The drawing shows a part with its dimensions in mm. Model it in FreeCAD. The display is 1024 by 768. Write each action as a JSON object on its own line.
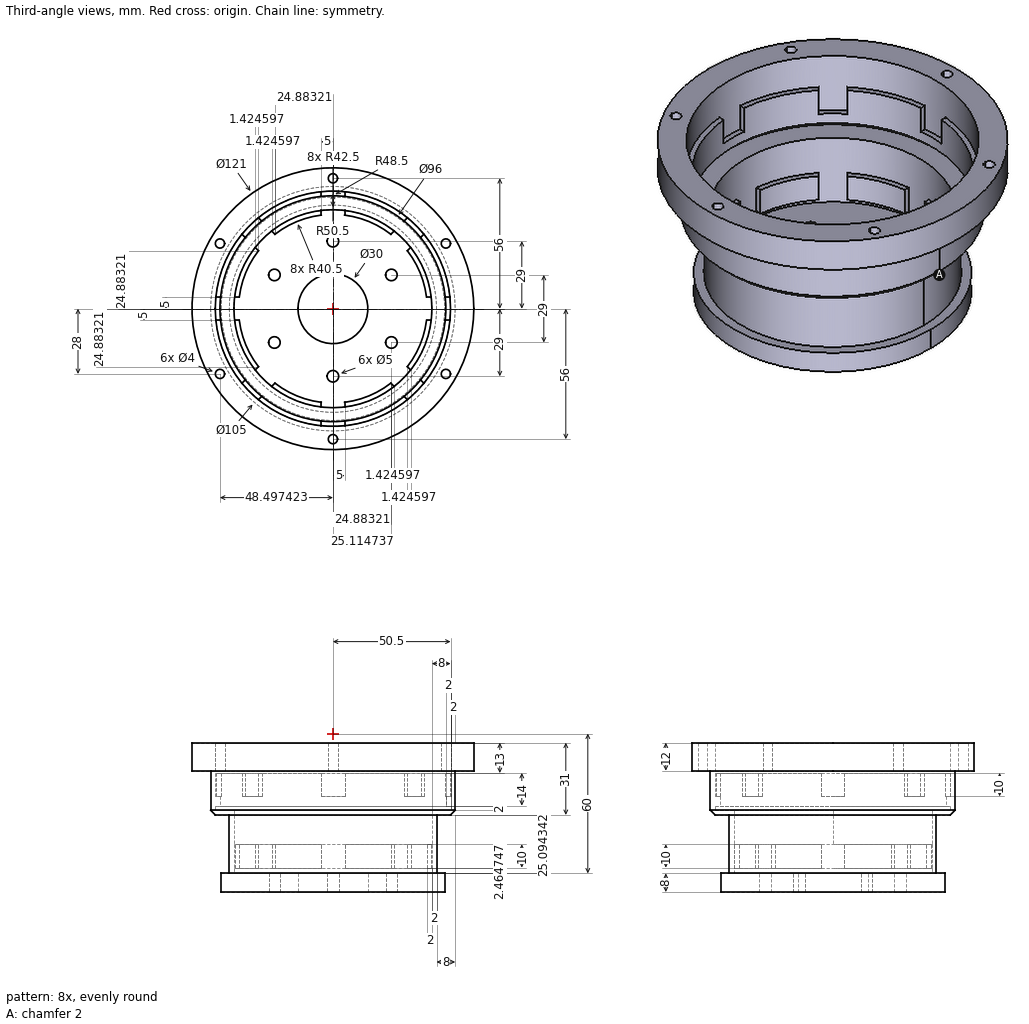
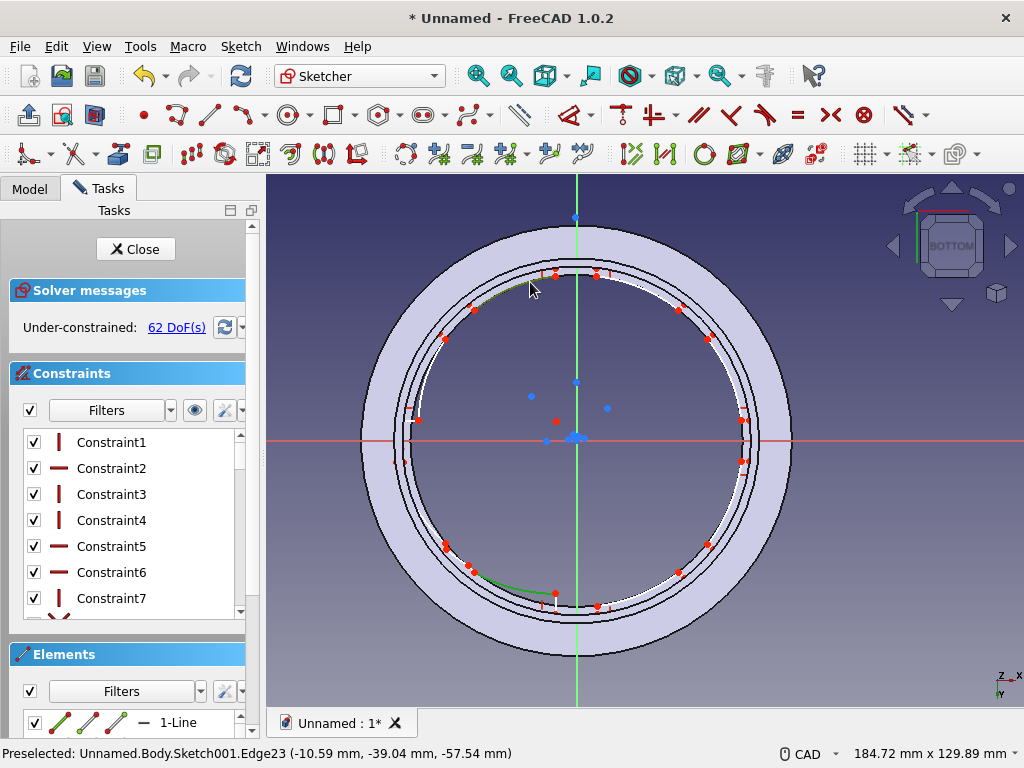
{"action": "left_click", "coordinate": [621, 116]}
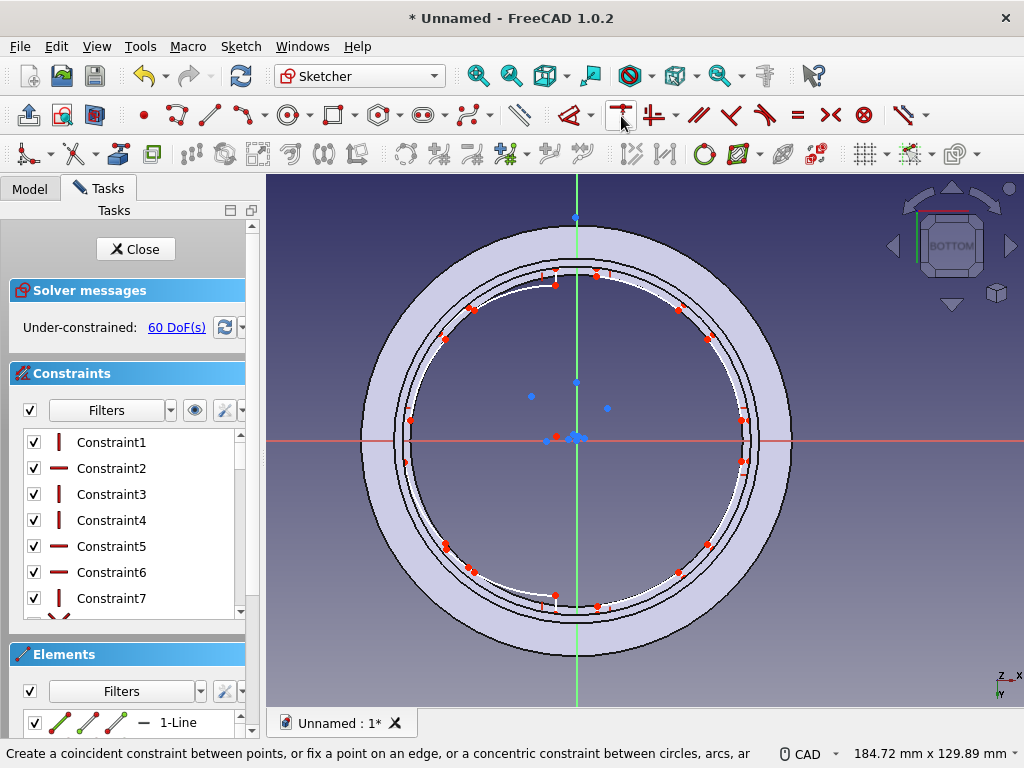
{"action": "left_click", "coordinate": [497, 584]}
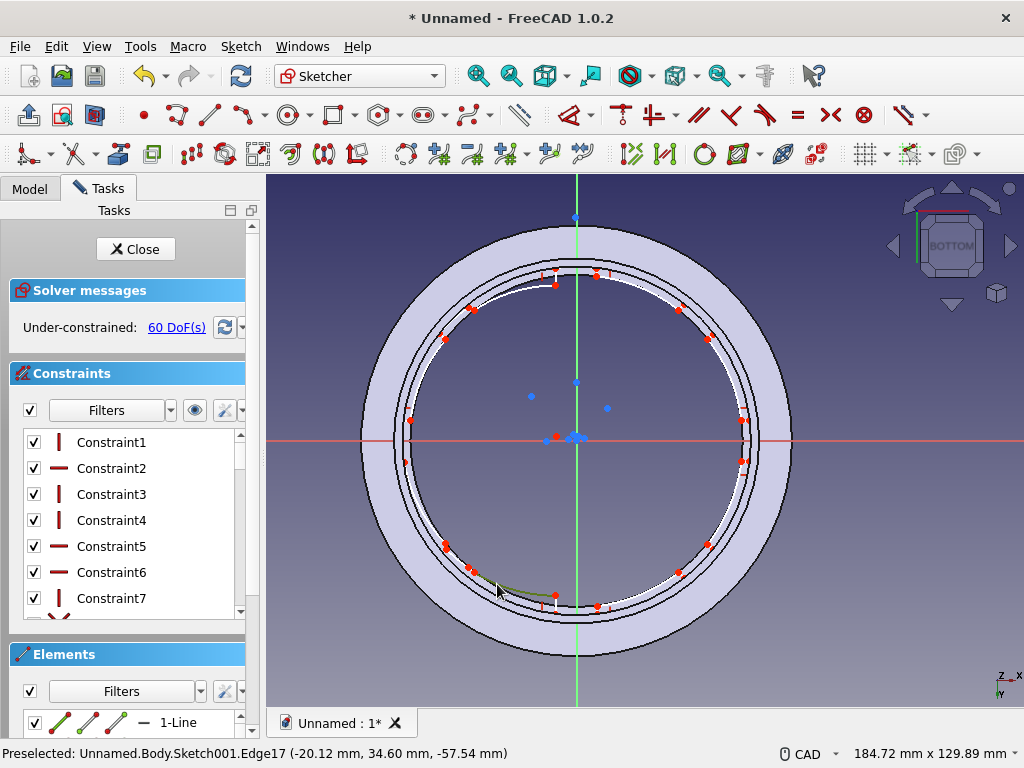
{"action": "left_click", "coordinate": [576, 267]}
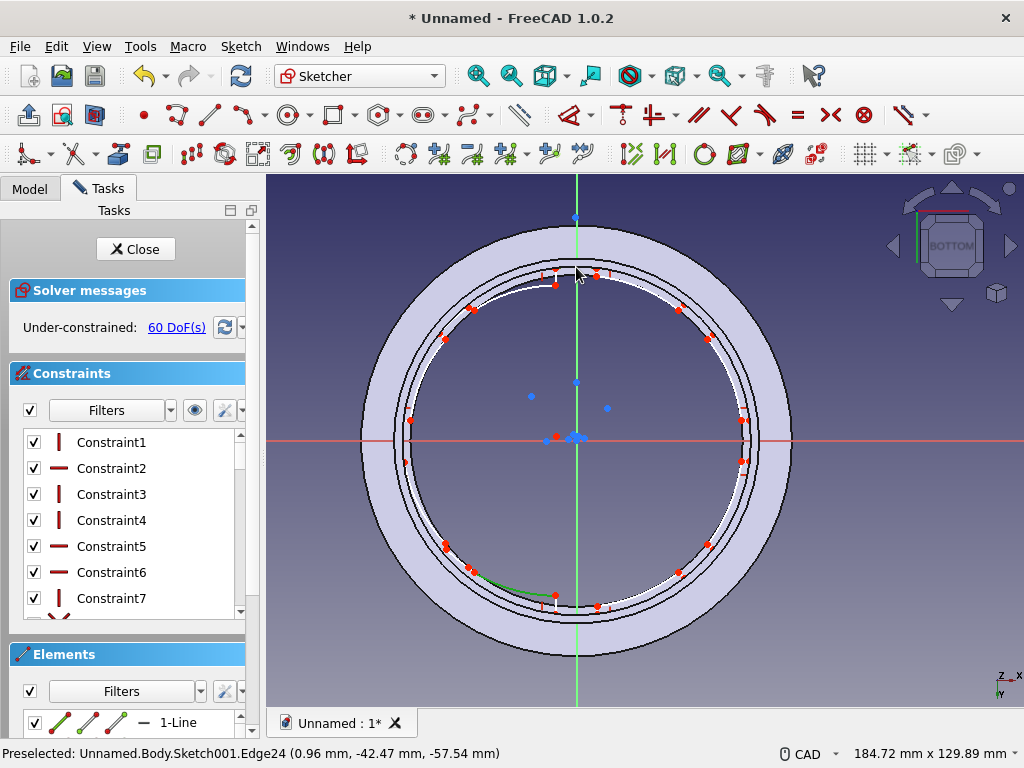
{"action": "left_click", "coordinate": [621, 116]}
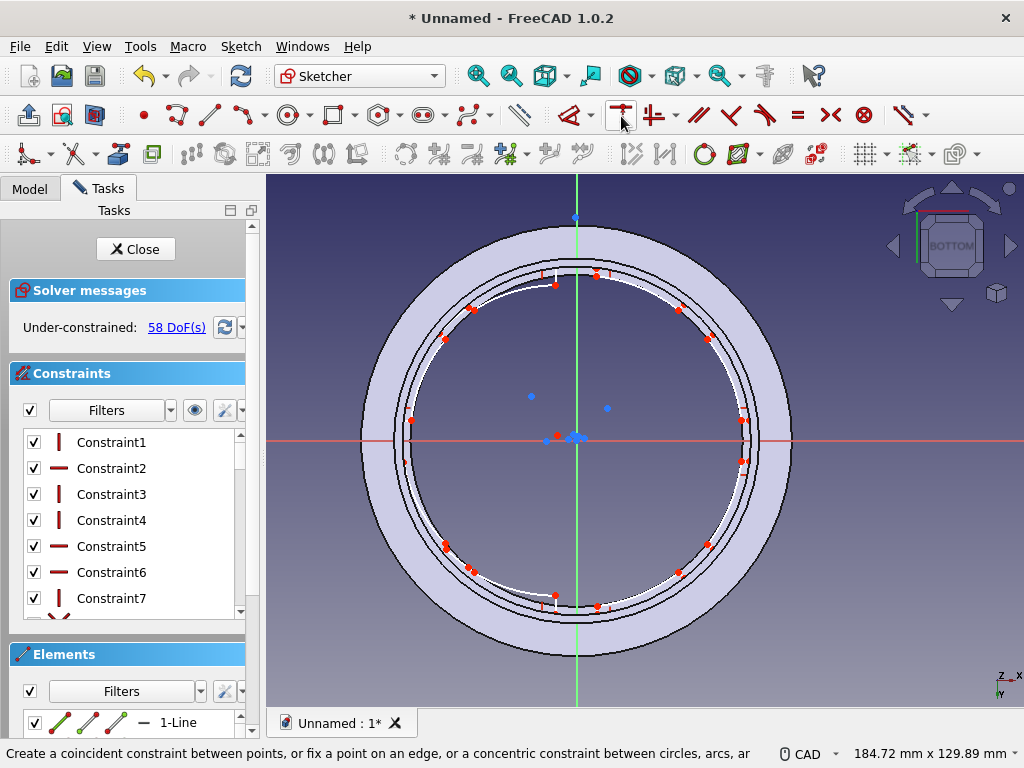
{"action": "left_click", "coordinate": [497, 584]}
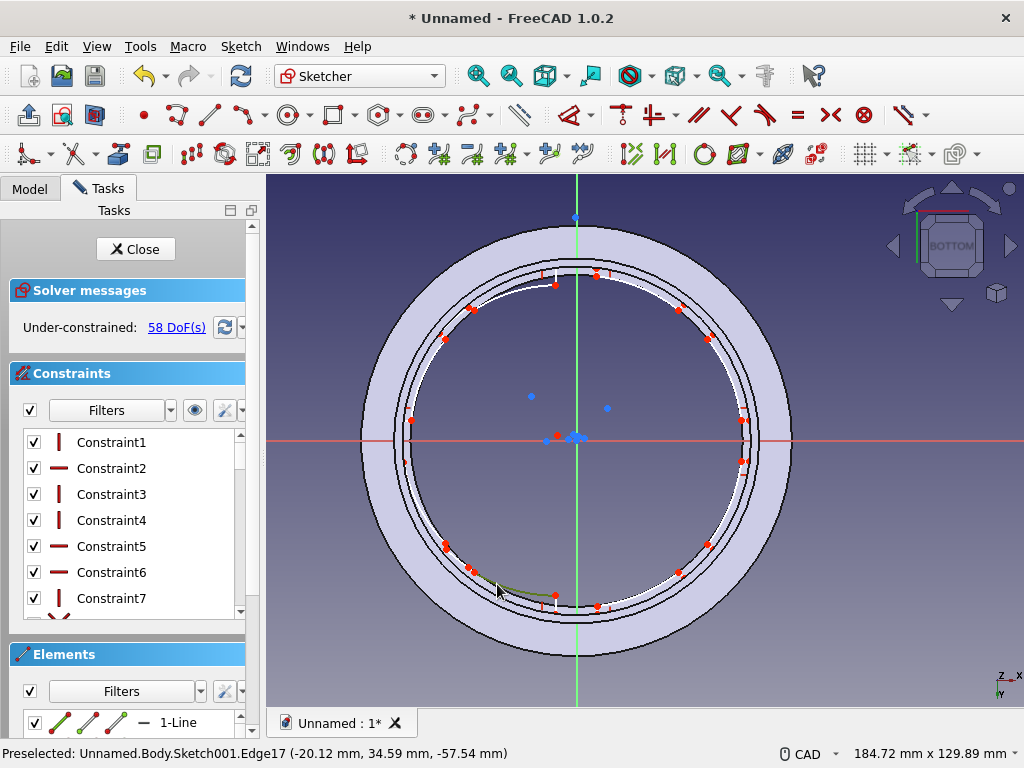
{"action": "left_click", "coordinate": [656, 295]}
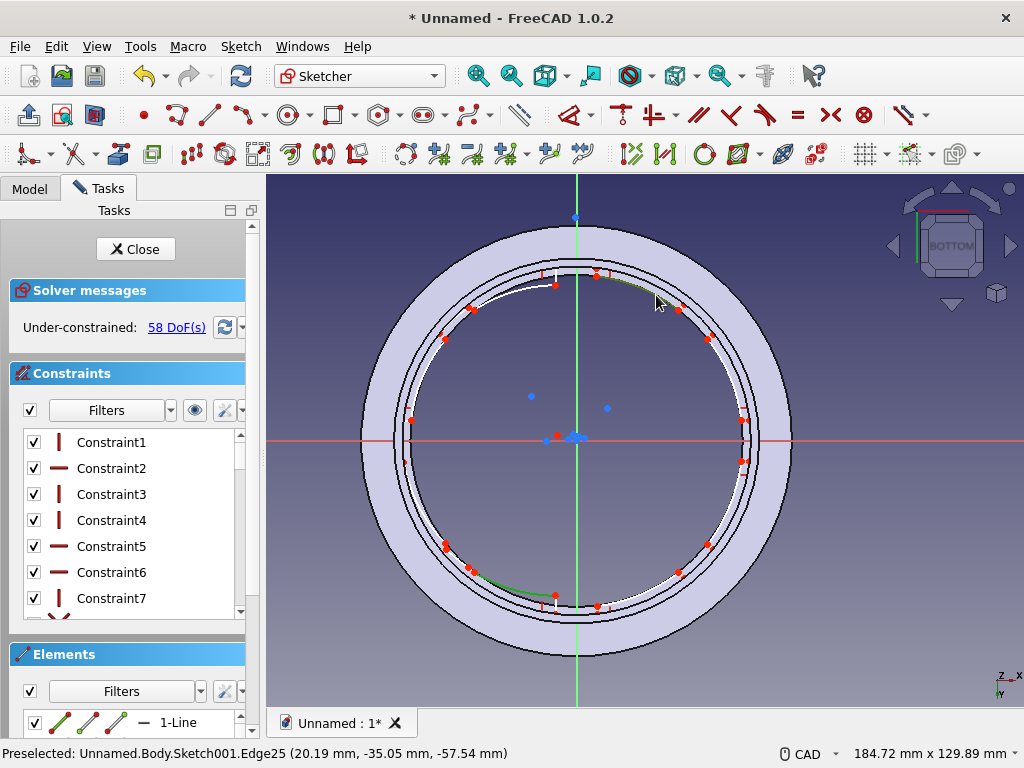
{"action": "key", "text": "c"}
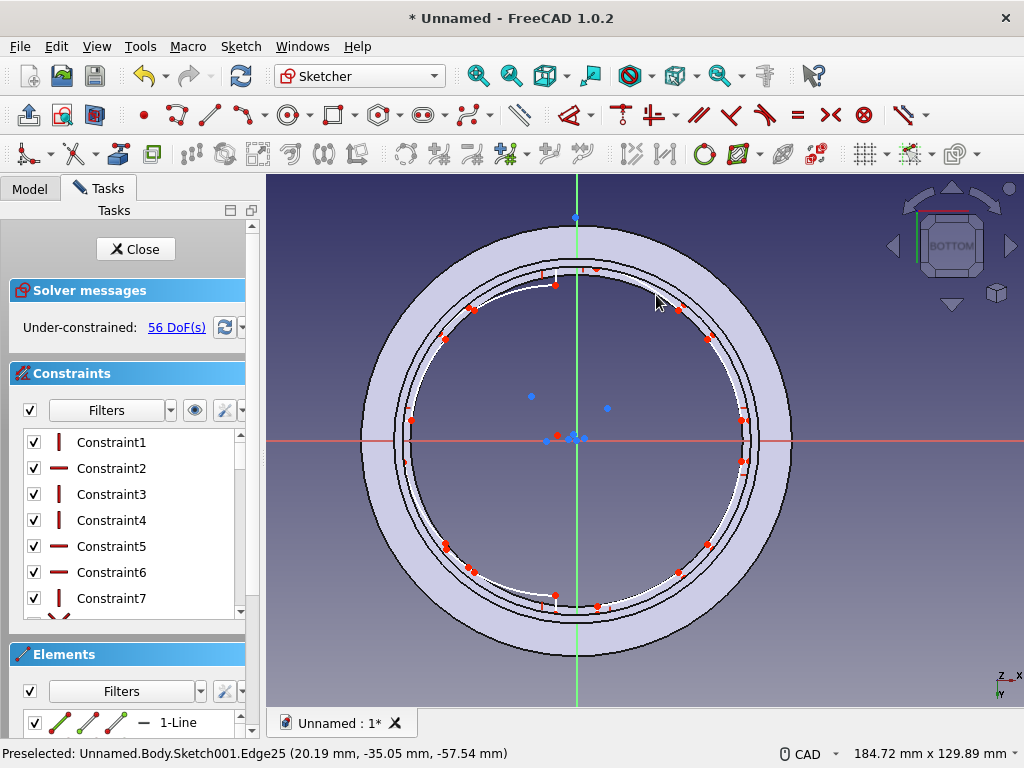
{"action": "left_click", "coordinate": [497, 584]}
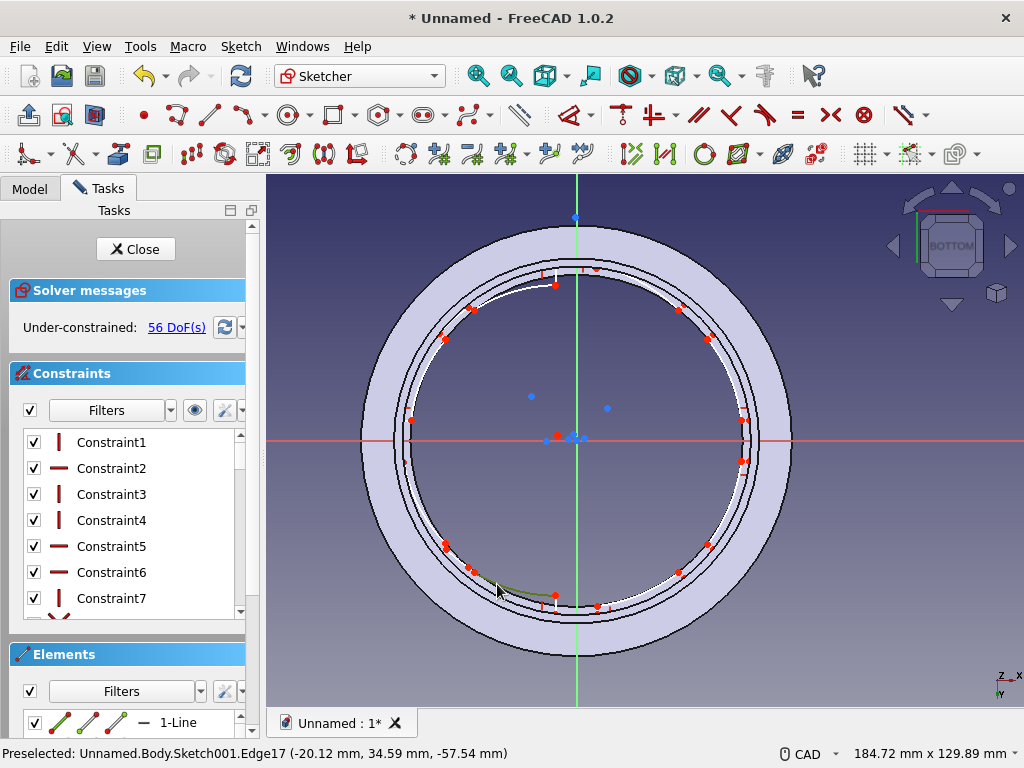
{"action": "left_click", "coordinate": [706, 324]}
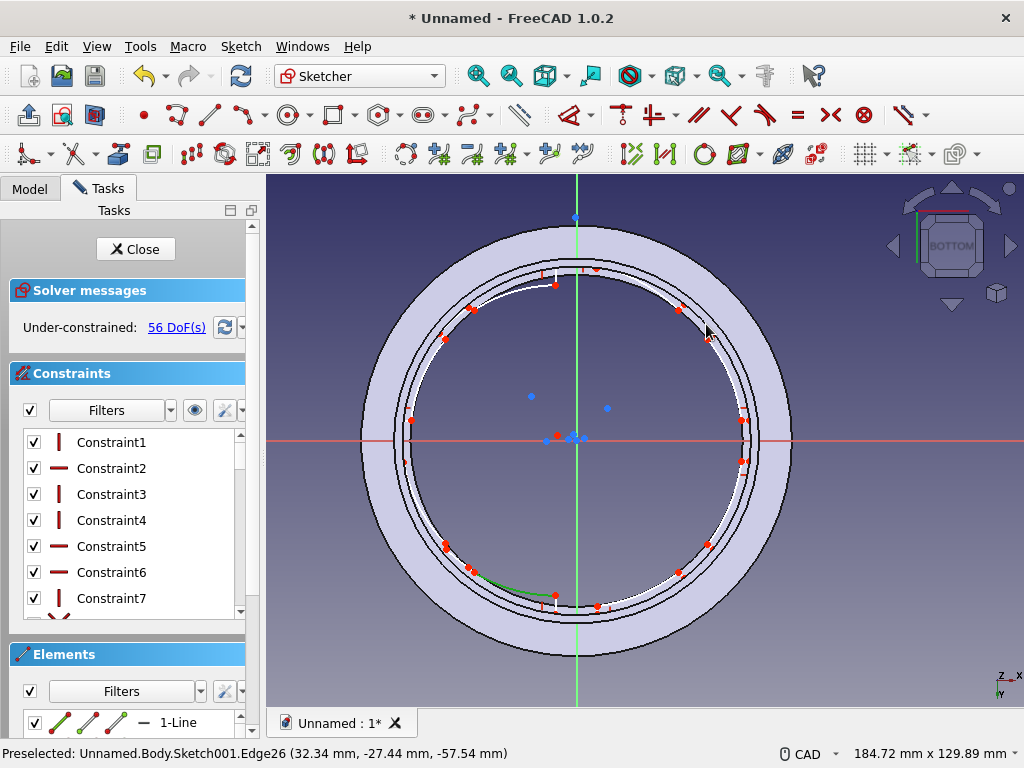
{"action": "key", "text": "c"}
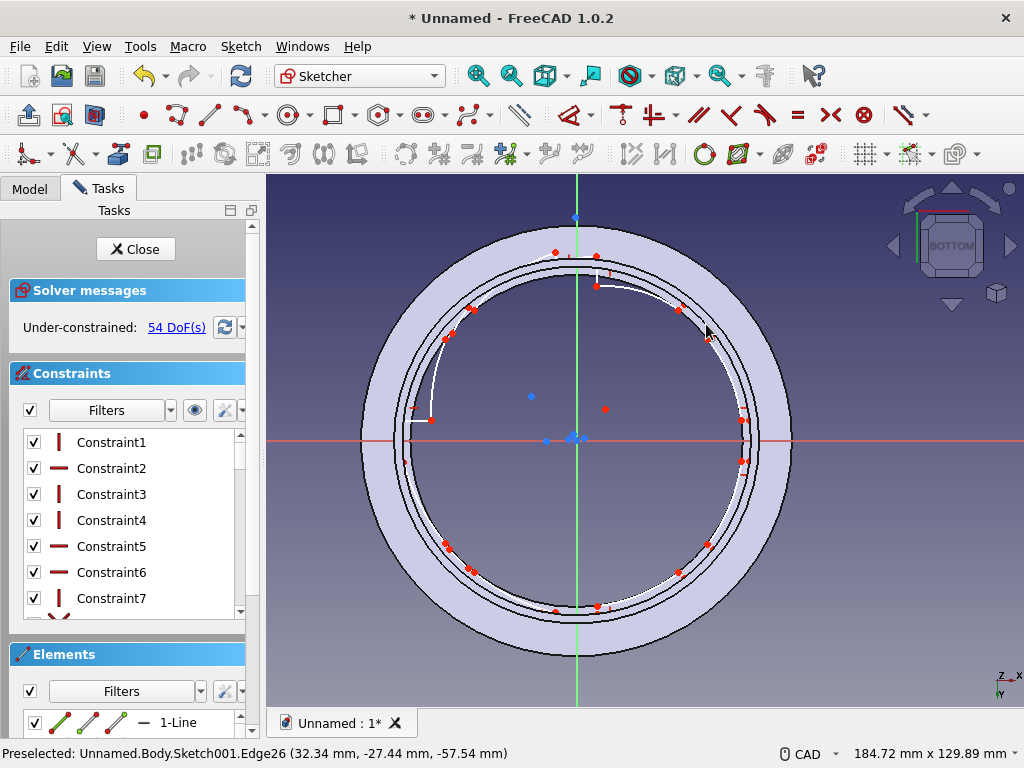
{"action": "left_click", "coordinate": [497, 588]}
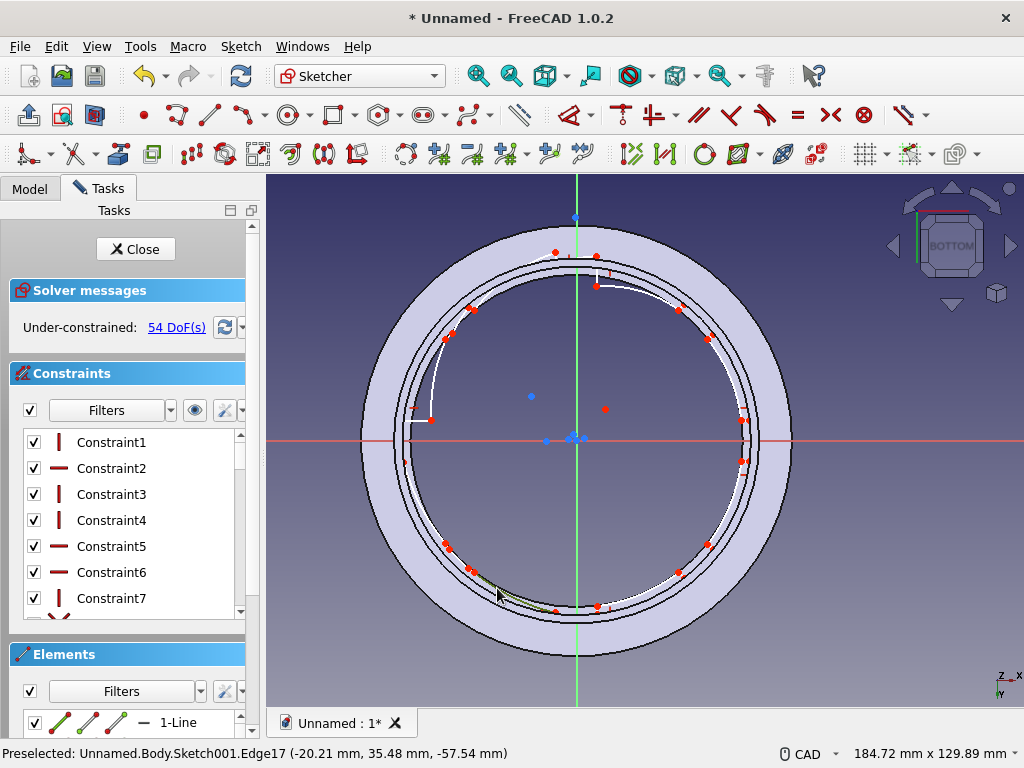
{"action": "left_click", "coordinate": [736, 395]}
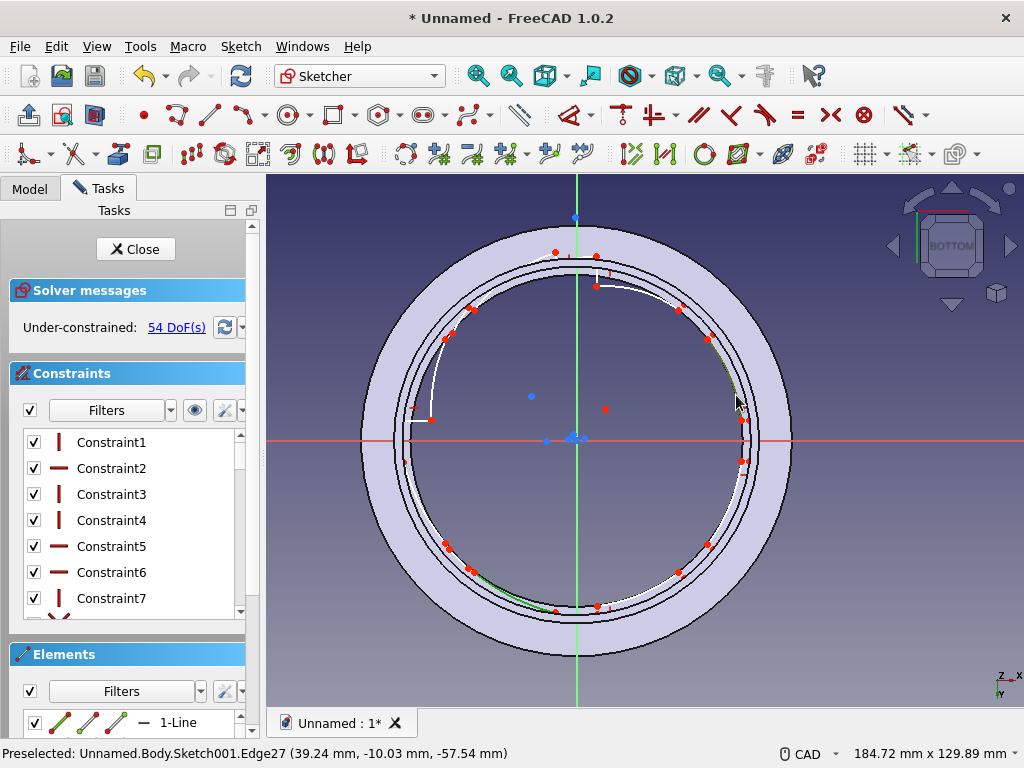
{"action": "left_click", "coordinate": [621, 116]}